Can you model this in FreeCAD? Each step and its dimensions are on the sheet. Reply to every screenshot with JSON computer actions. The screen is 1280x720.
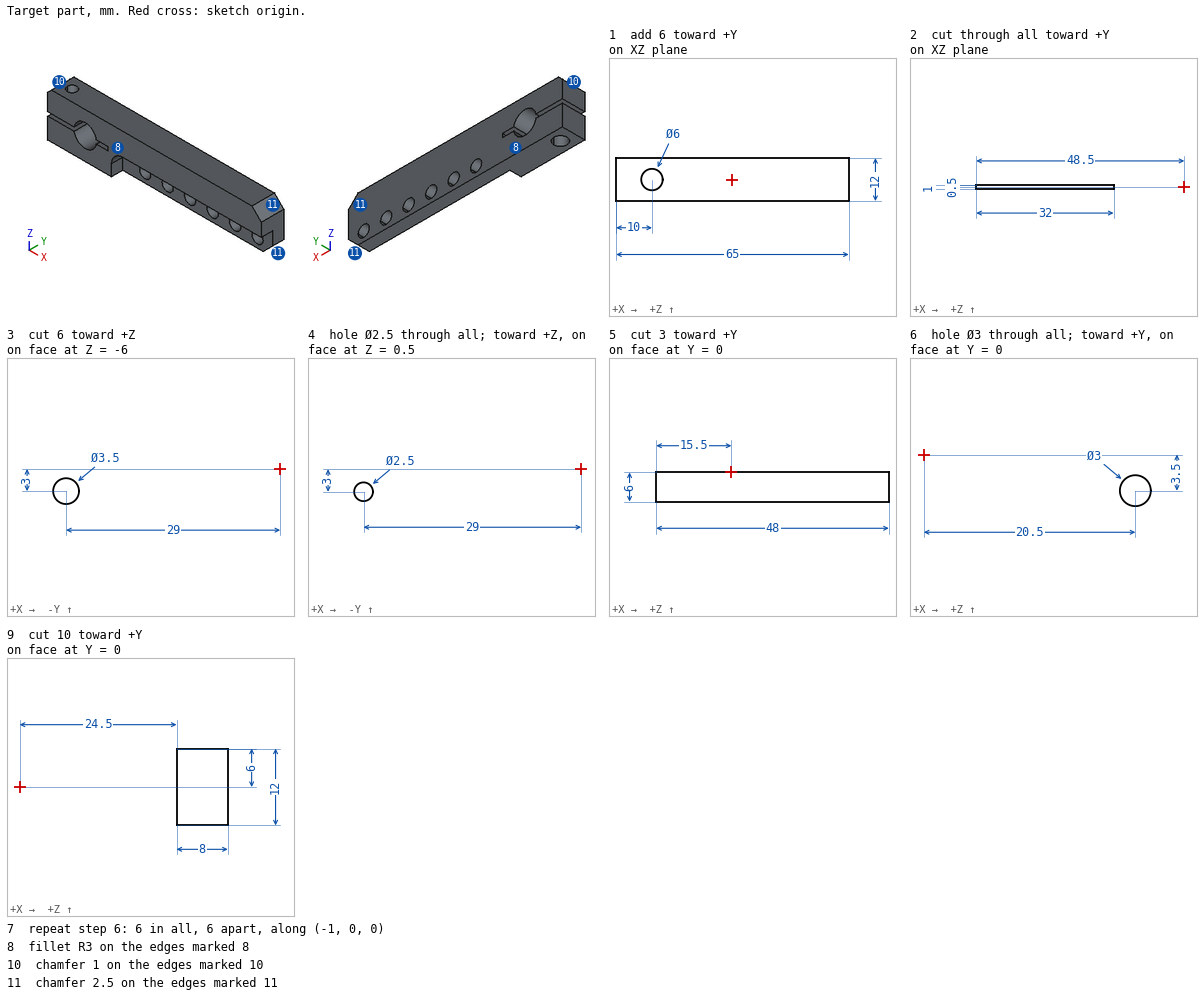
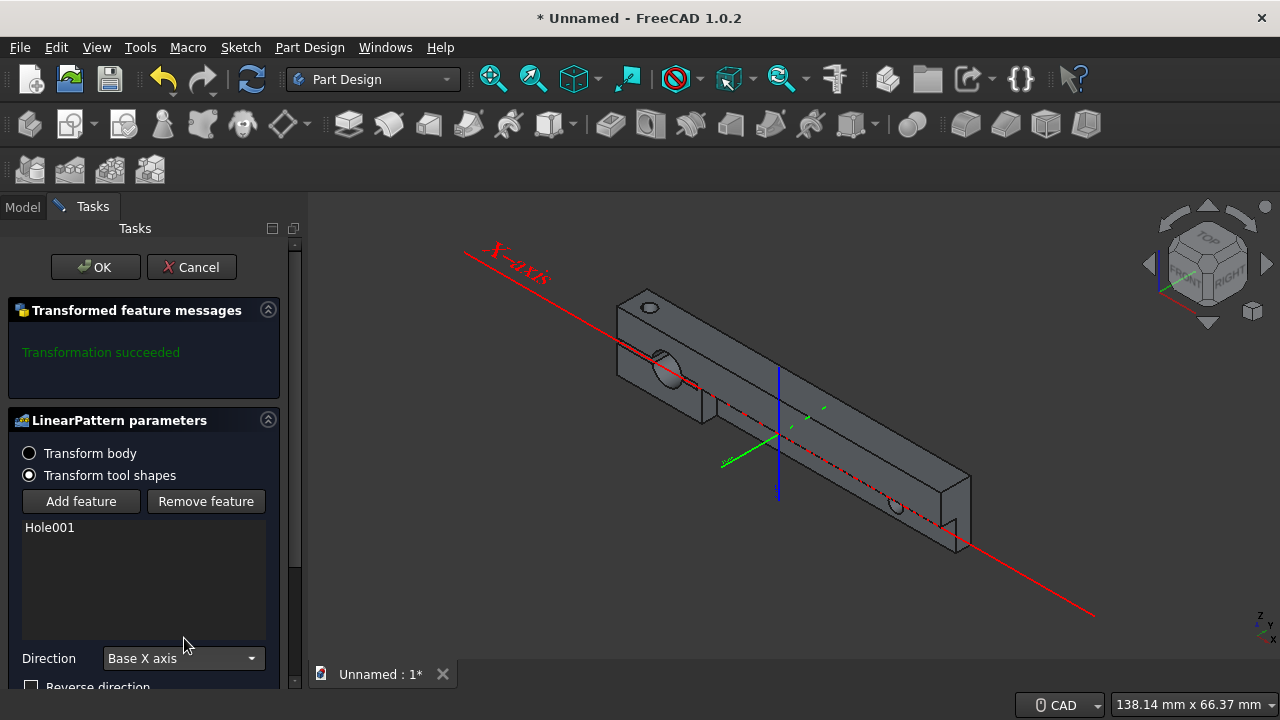
{"action": "scroll", "coordinate": [295, 463], "scroll_direction": "down", "scroll_amount": 2}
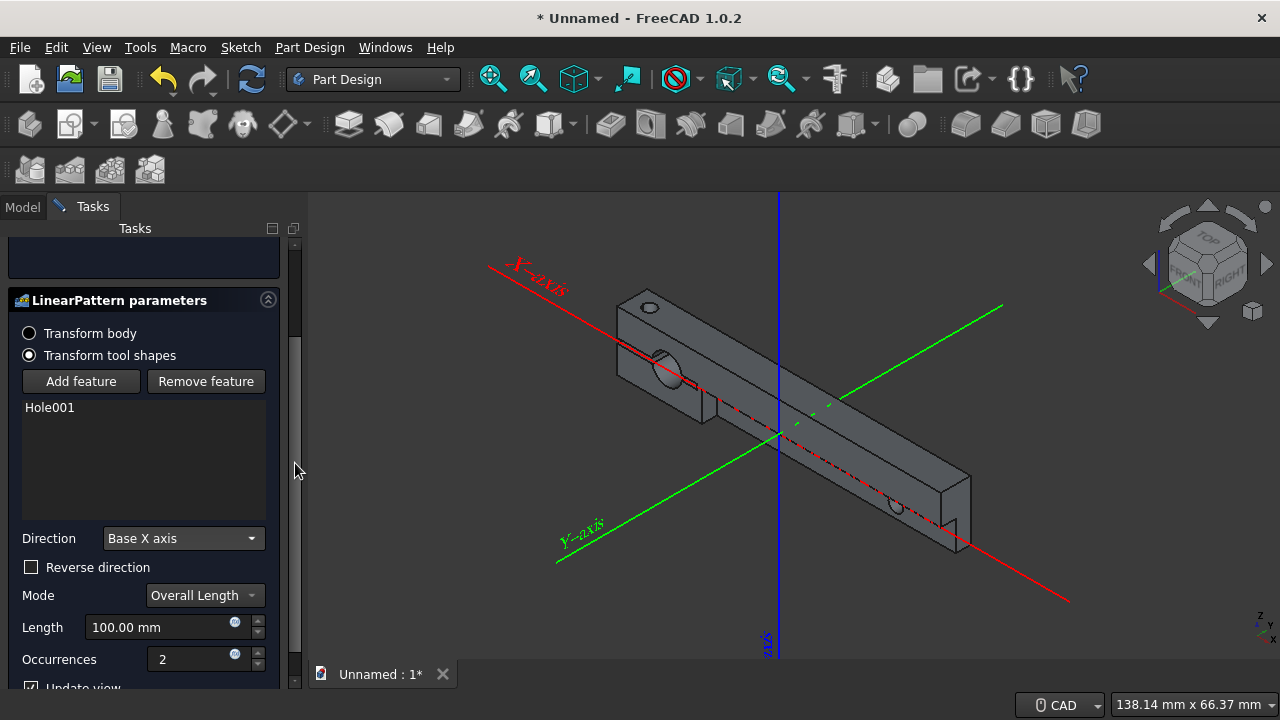
{"action": "left_click", "coordinate": [206, 596]}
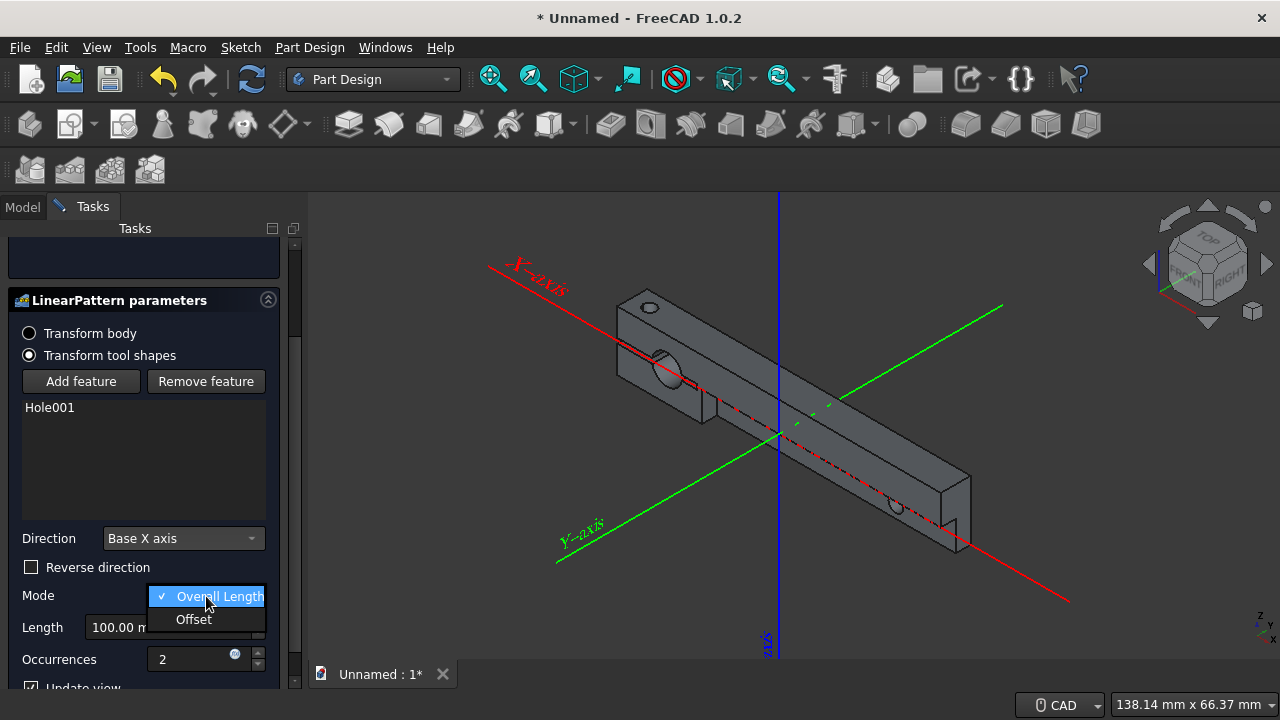
{"action": "left_click", "coordinate": [206, 620]}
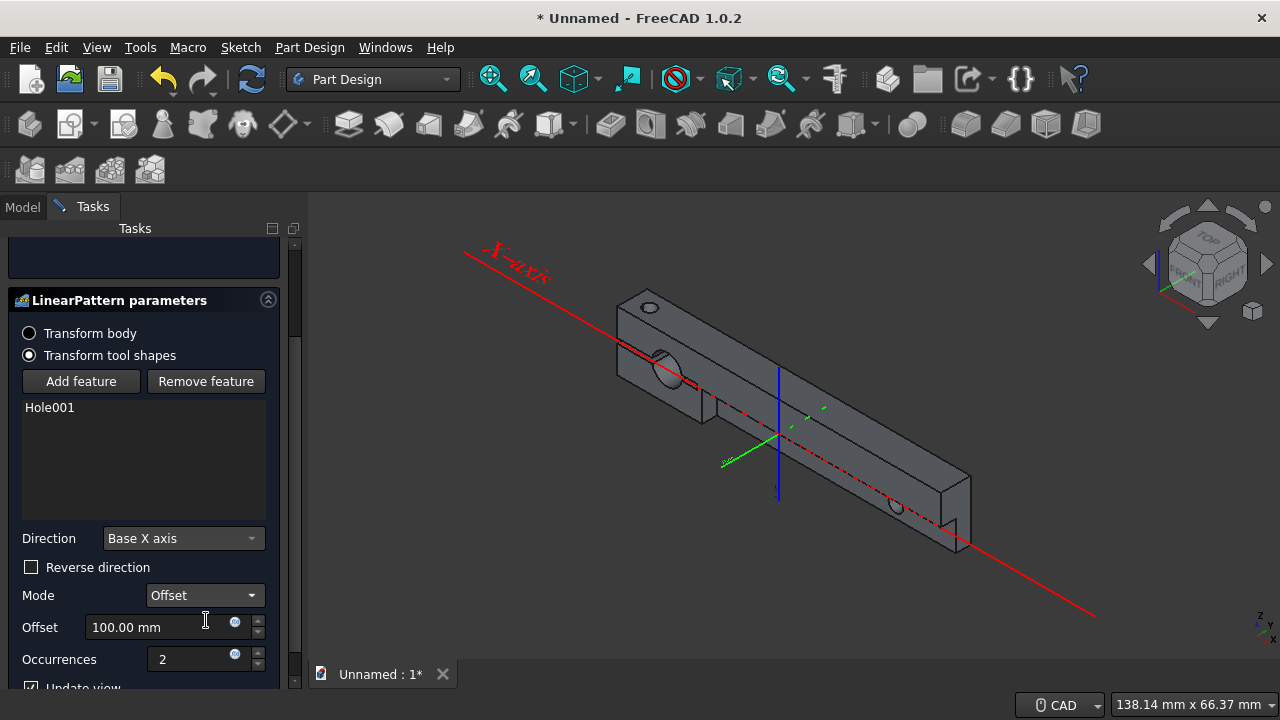
{"action": "triple_click", "coordinate": [168, 627]}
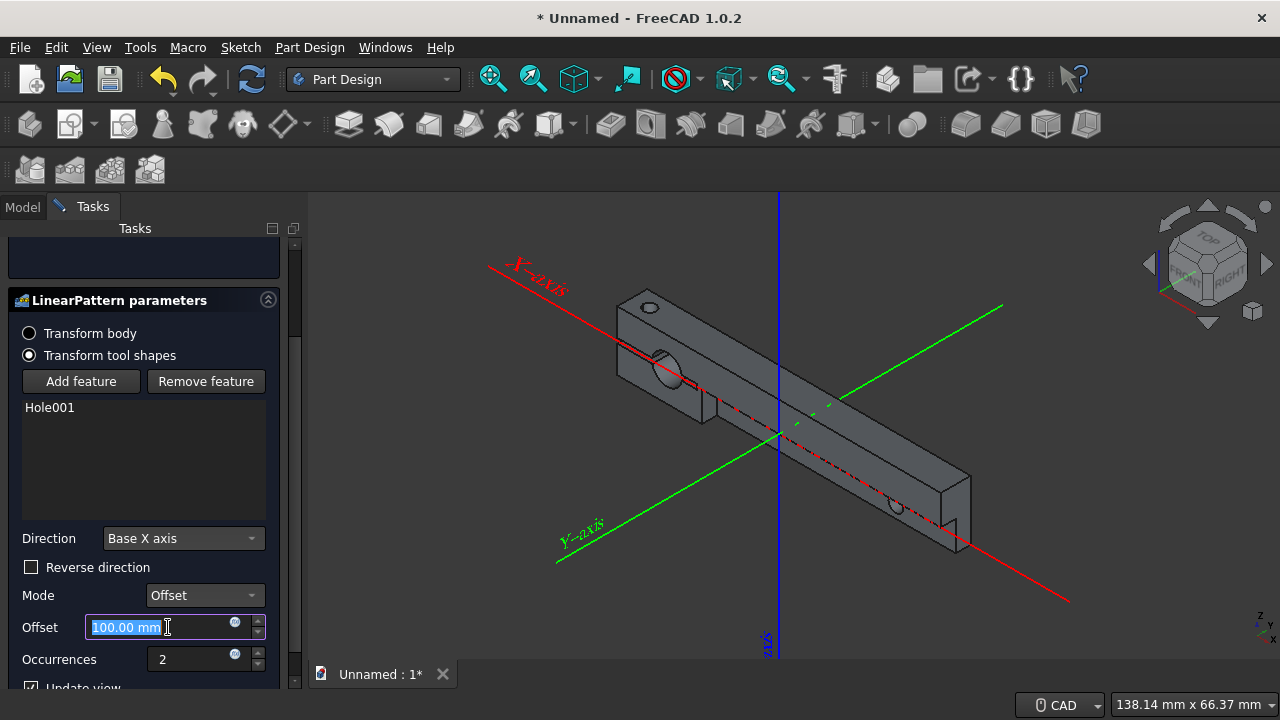
{"action": "type", "text": "6"}
{"action": "key", "text": "Tab"}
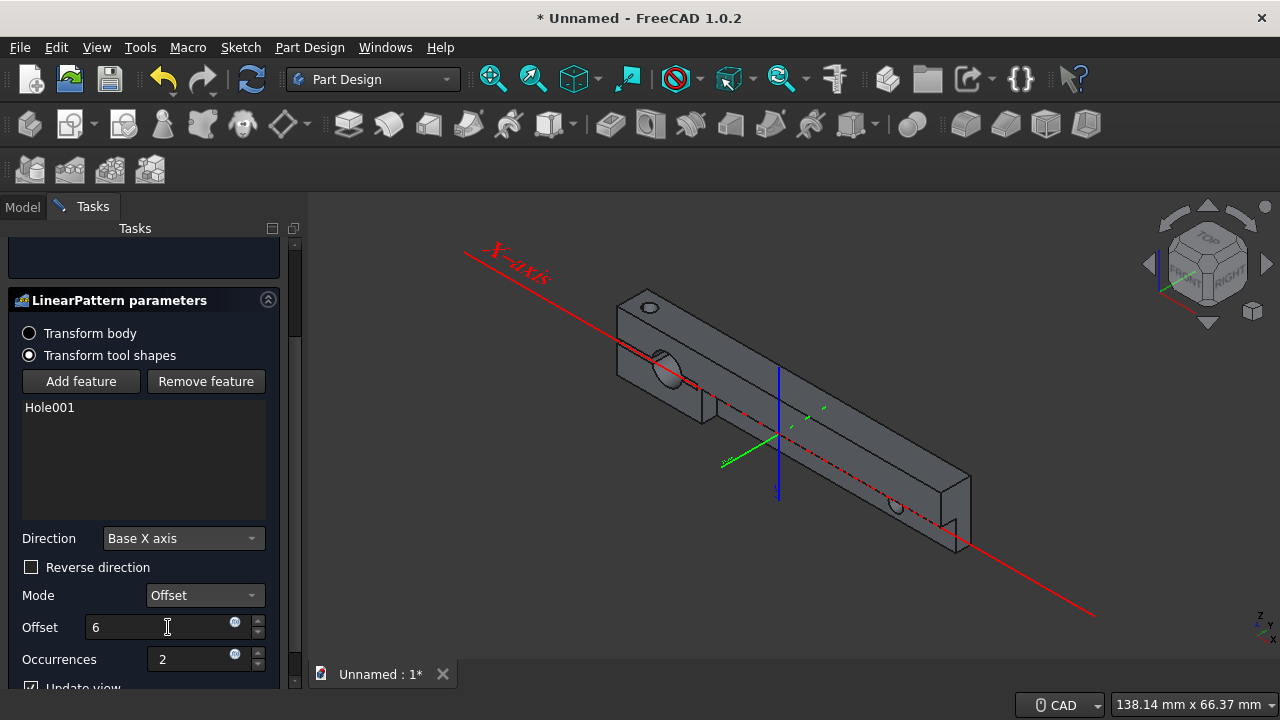
{"action": "triple_click", "coordinate": [198, 659]}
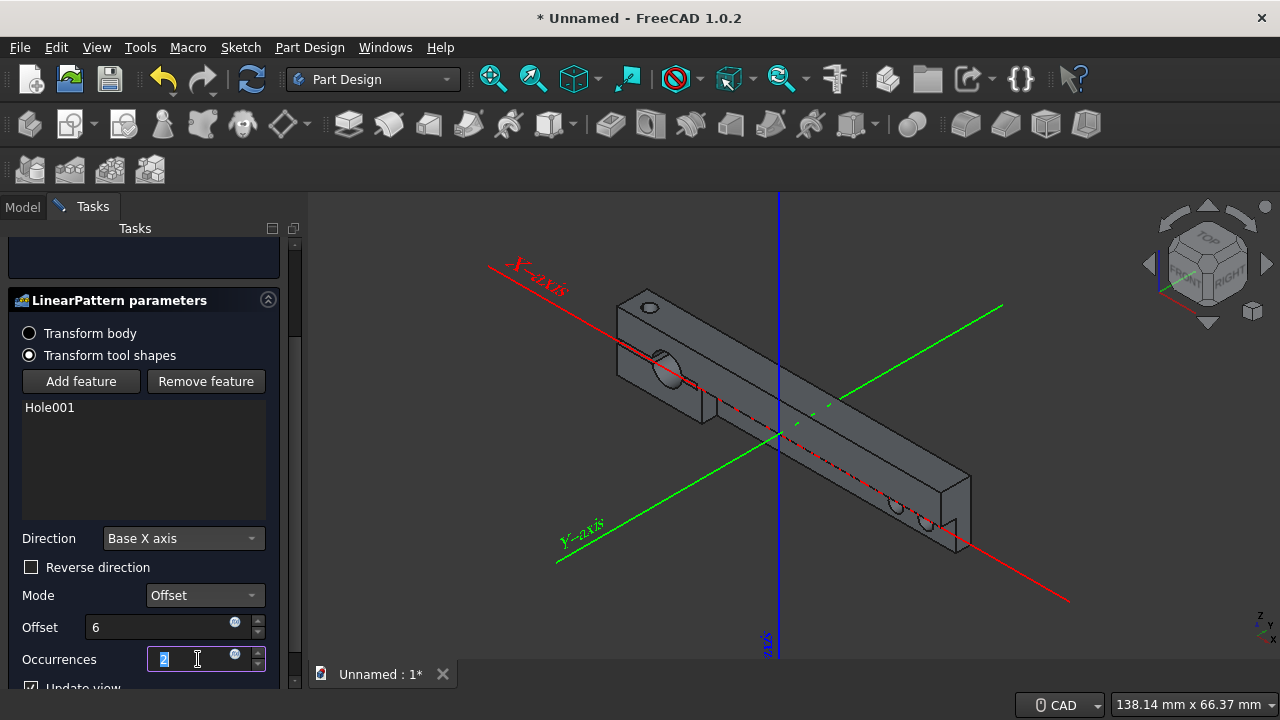
{"action": "type", "text": "6"}
{"action": "key", "text": "Tab"}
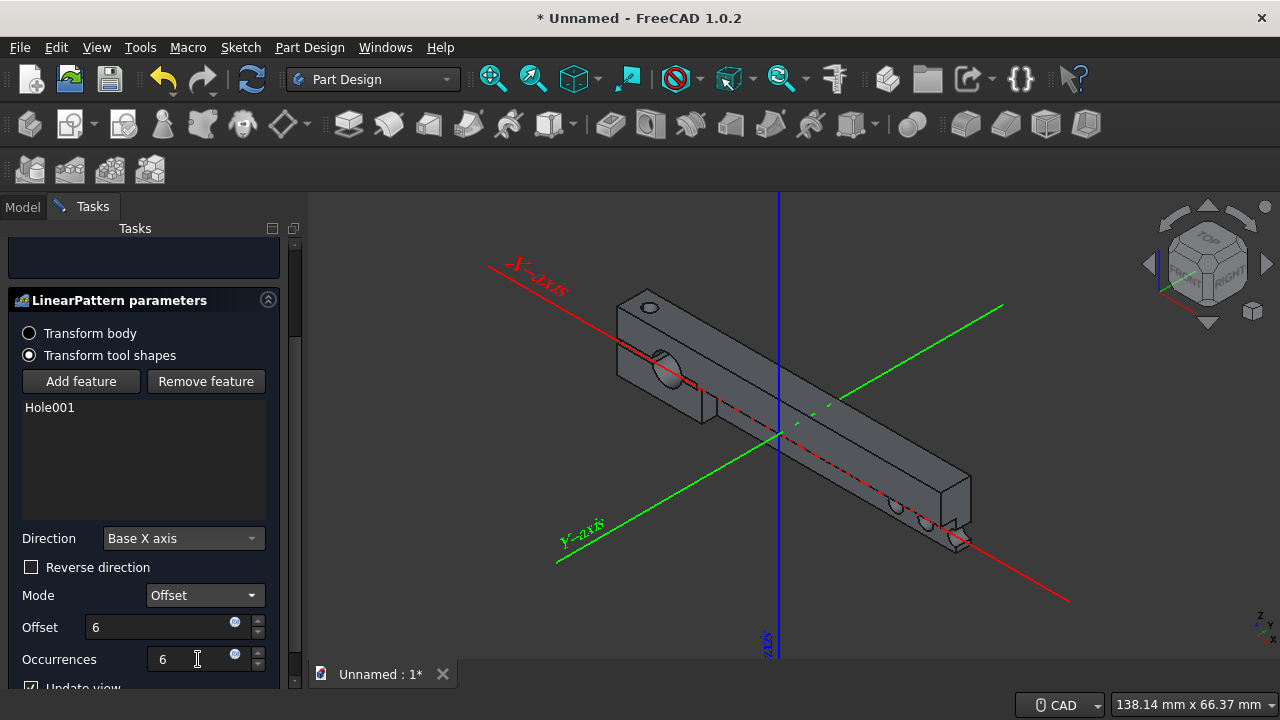
{"action": "left_click", "coordinate": [30, 567]}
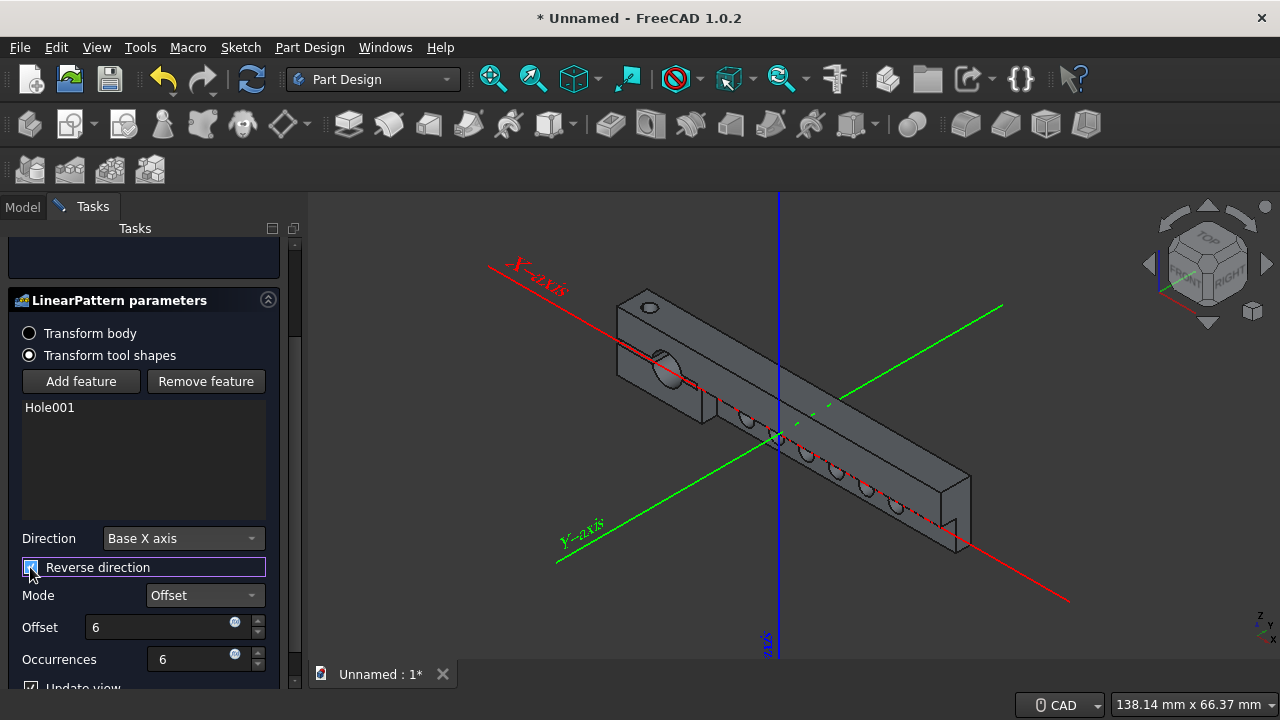
{"action": "scroll", "coordinate": [295, 463], "scroll_direction": "up", "scroll_amount": 3}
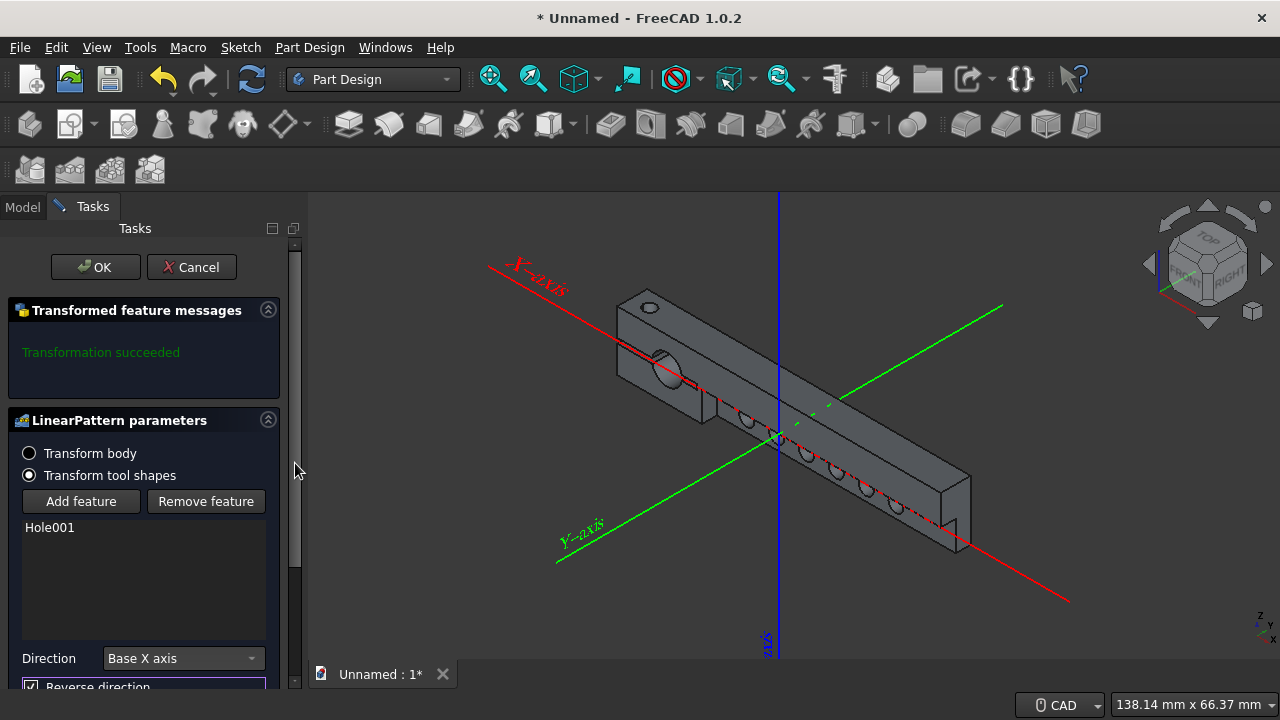
{"action": "left_click", "coordinate": [96, 267]}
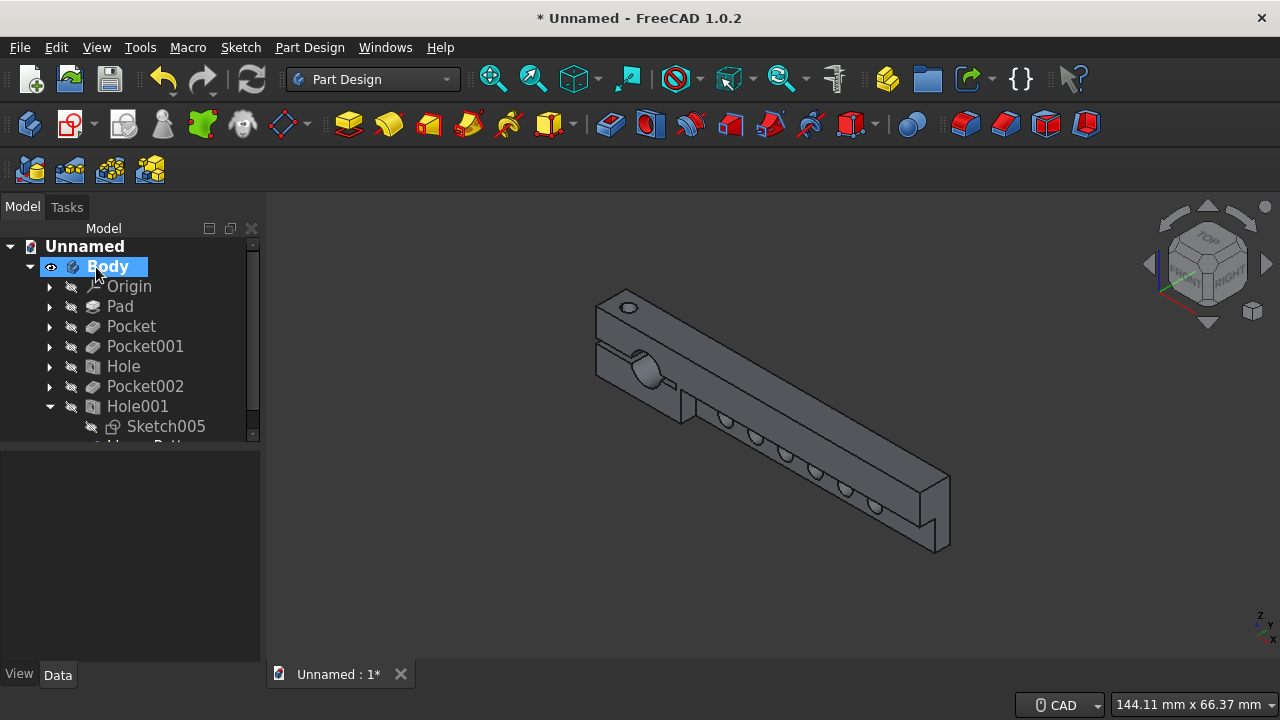
{"action": "scroll", "coordinate": [688, 384], "scroll_direction": "up", "scroll_amount": 4}